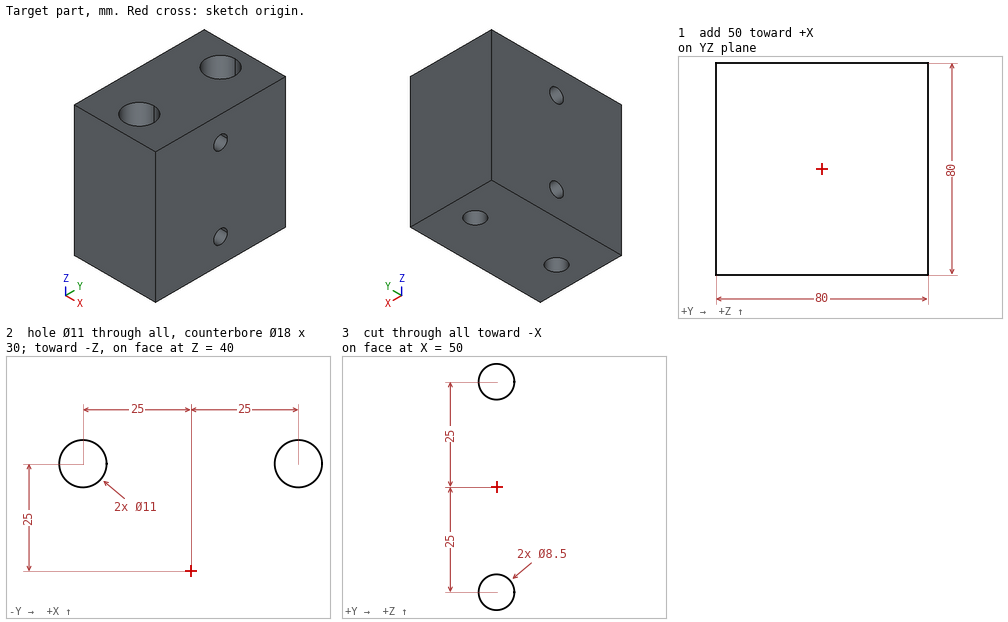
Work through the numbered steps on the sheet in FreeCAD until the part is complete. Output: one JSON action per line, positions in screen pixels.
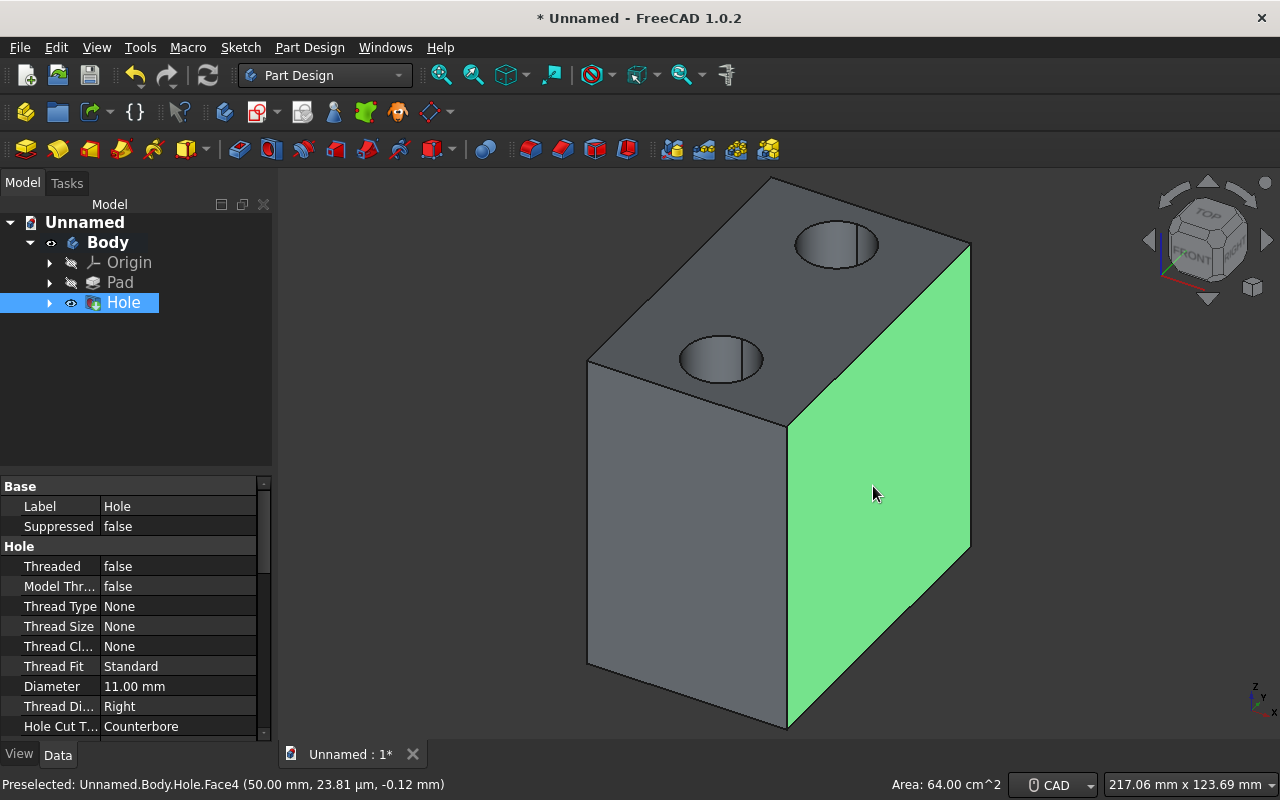
{"action": "left_click", "coordinate": [258, 112]}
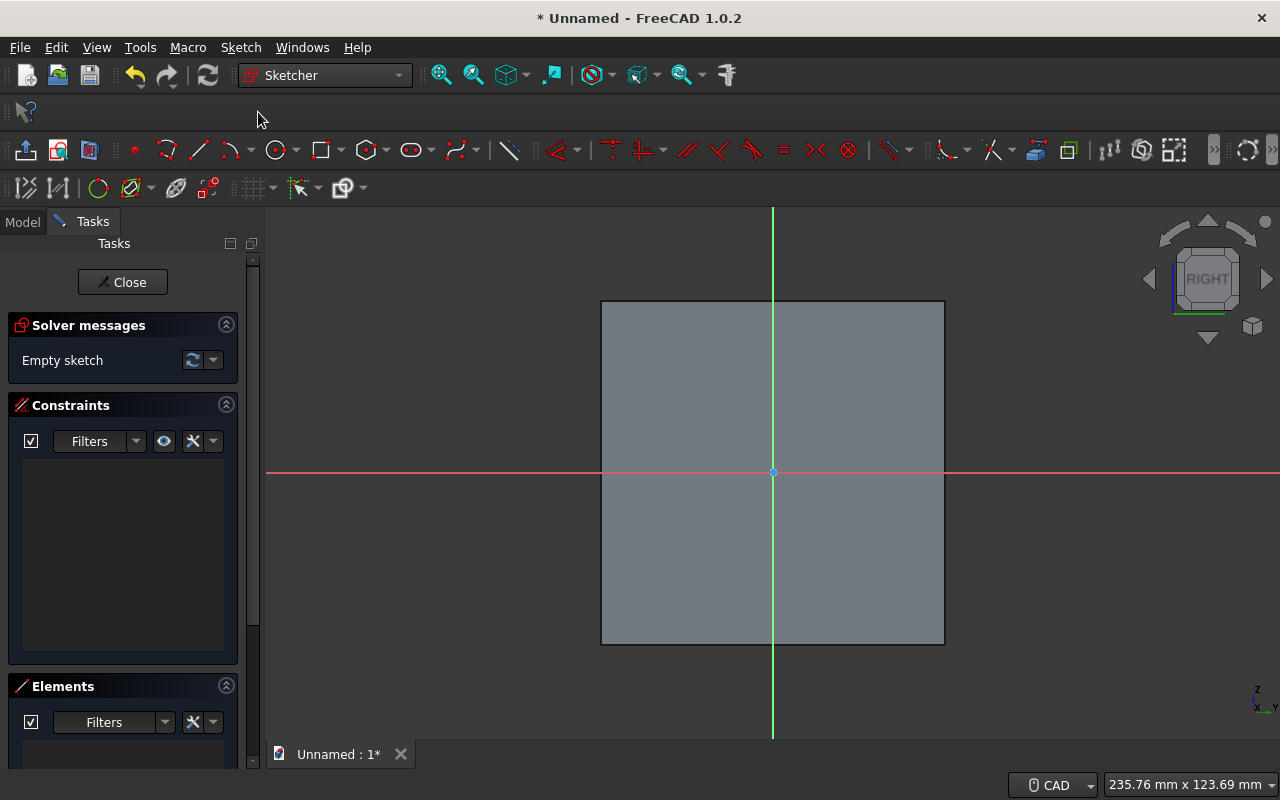
{"action": "left_click", "coordinate": [276, 150]}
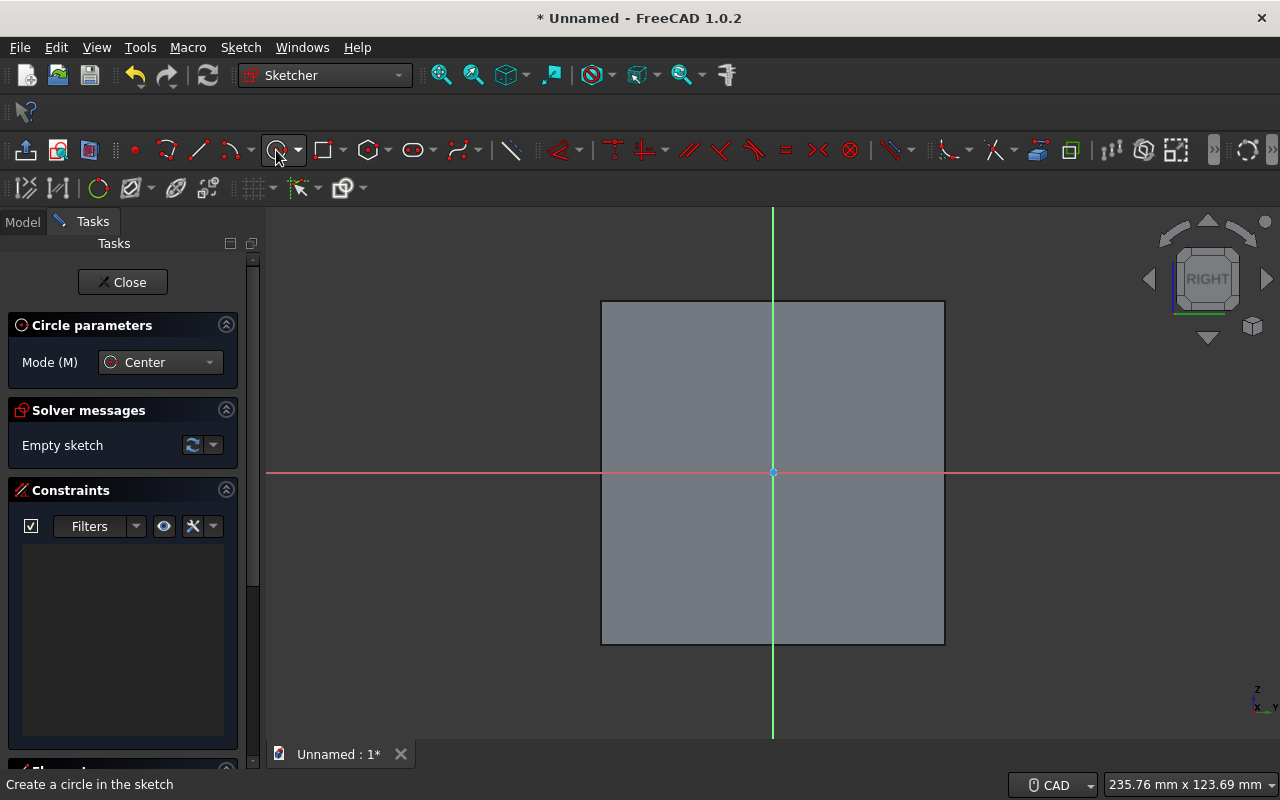
{"action": "scroll", "coordinate": [773, 581], "scroll_direction": "up", "scroll_amount": 2}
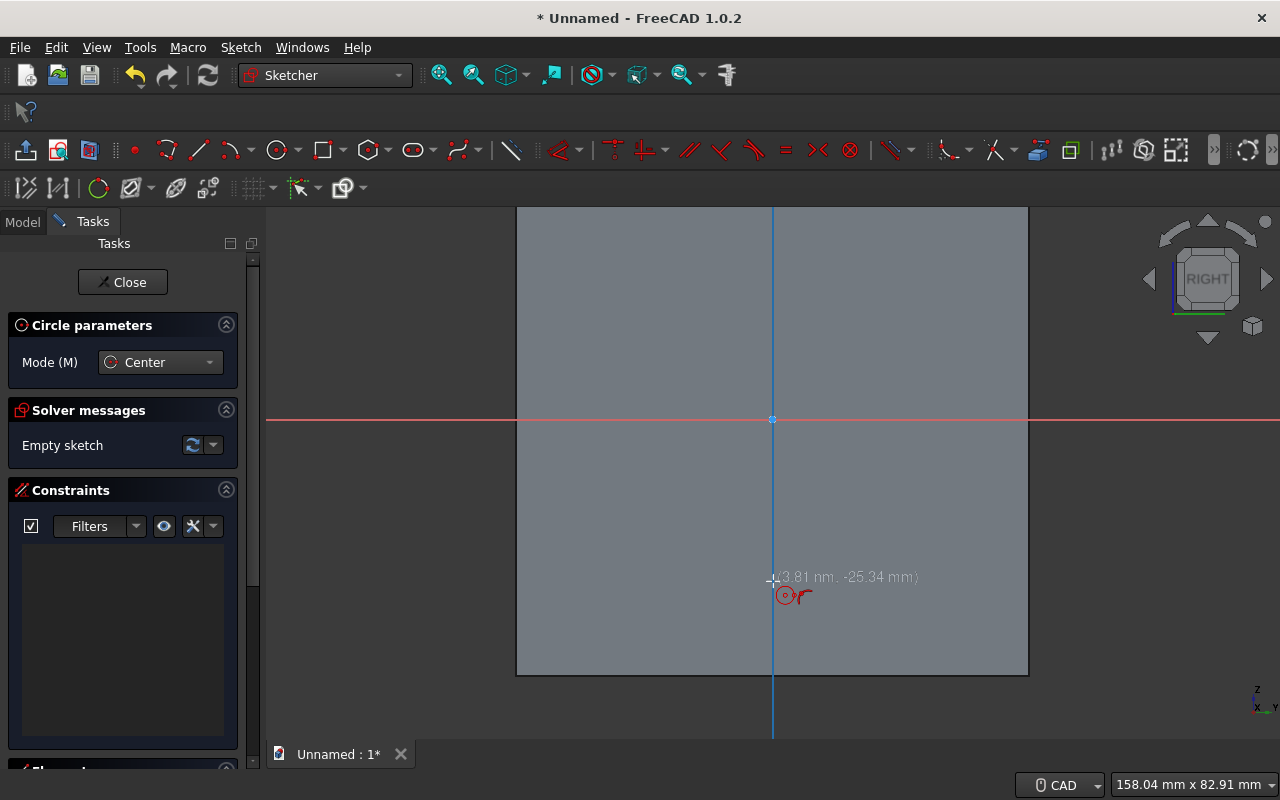
{"action": "left_click", "coordinate": [773, 580]}
{"action": "left_click", "coordinate": [792, 561]}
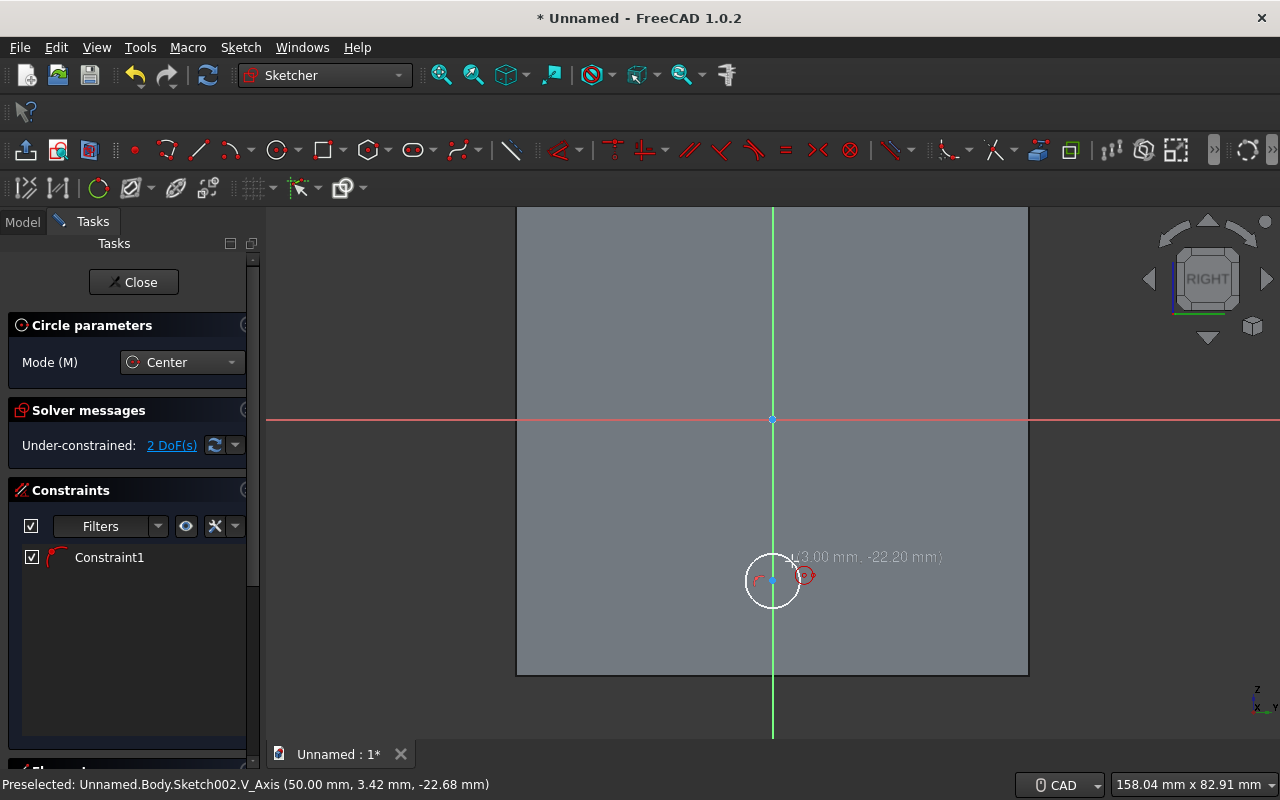
{"action": "left_click", "coordinate": [773, 259]}
{"action": "left_click", "coordinate": [792, 240]}
{"action": "key", "text": "Escape"}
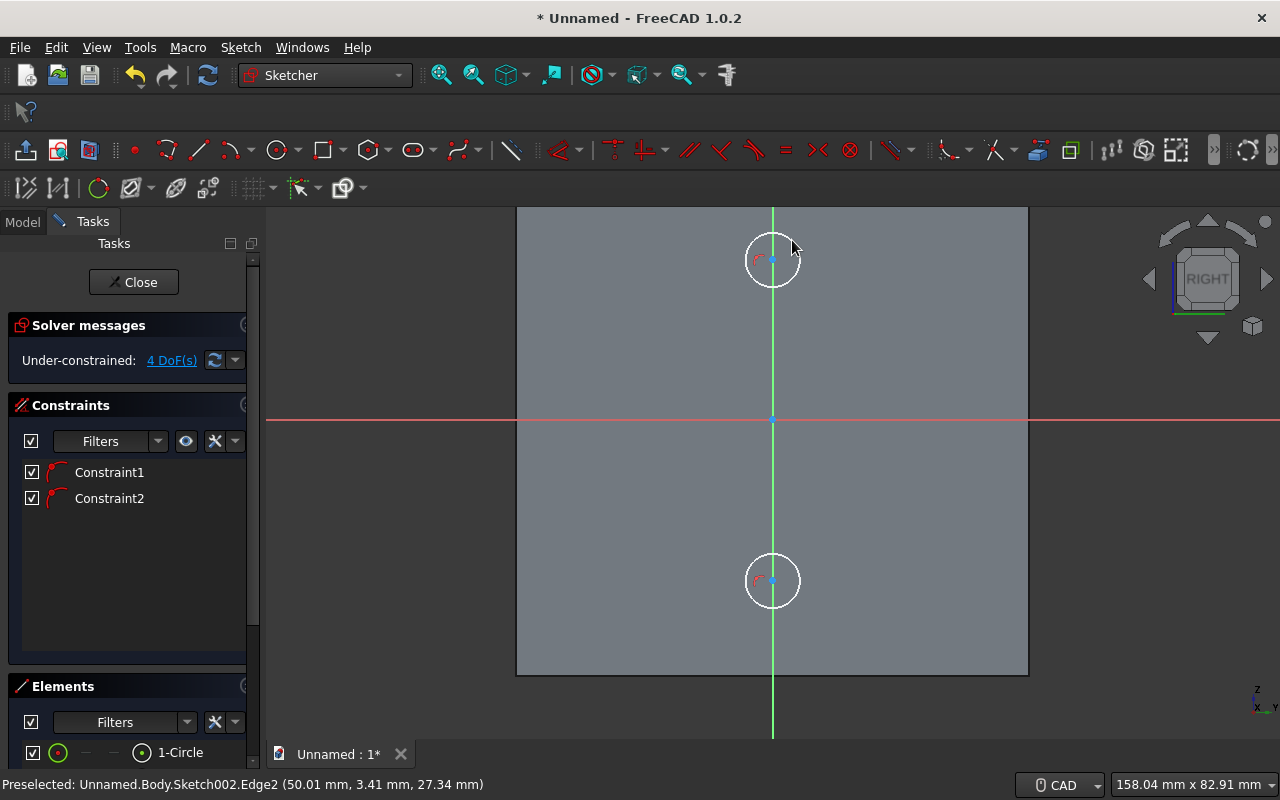
{"action": "left_click", "coordinate": [792, 562]}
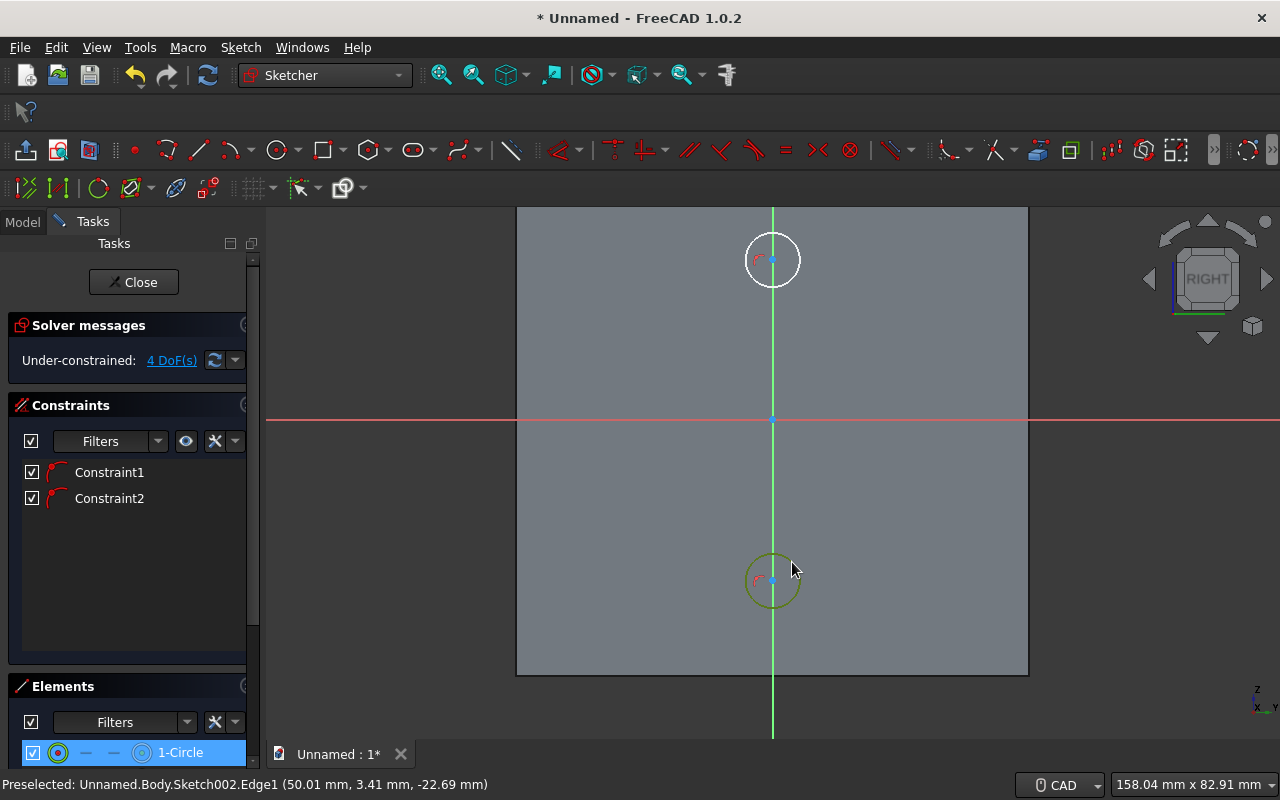
{"action": "left_click", "coordinate": [792, 241]}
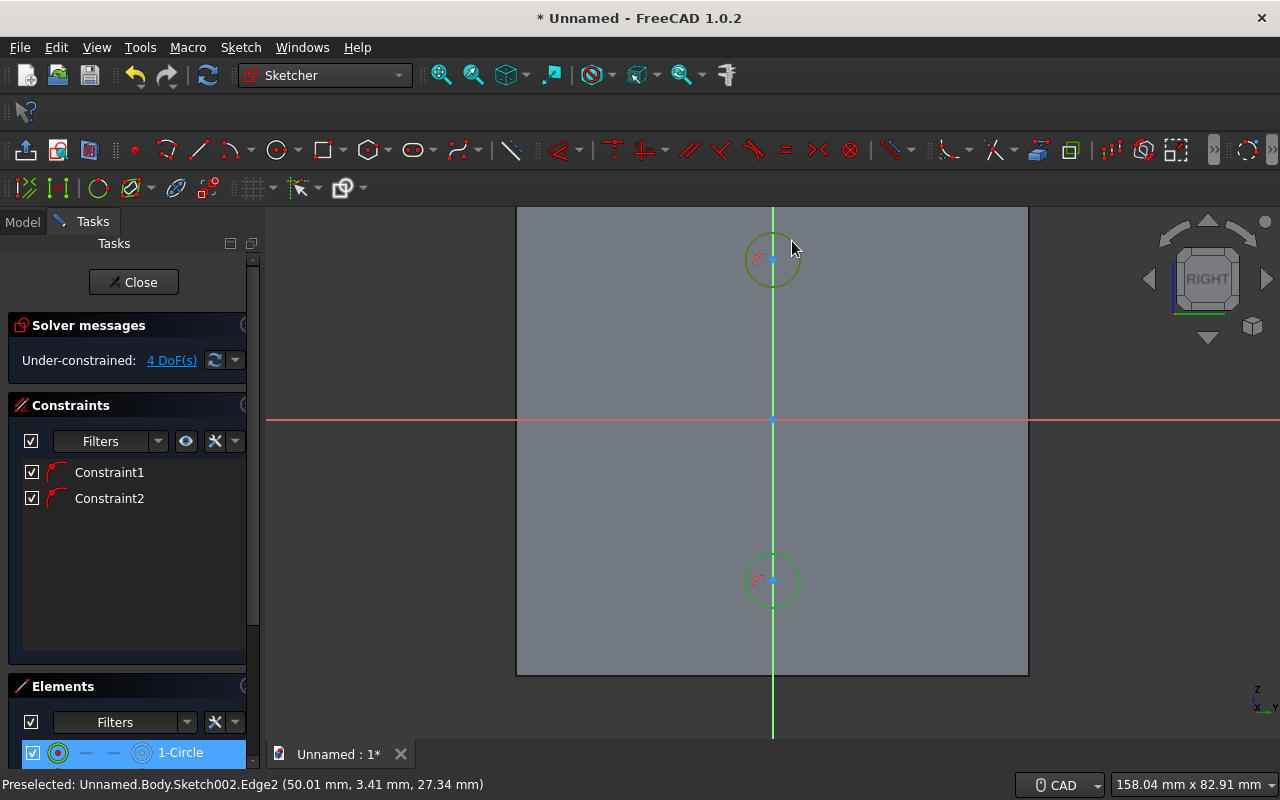
{"action": "left_click", "coordinate": [786, 150]}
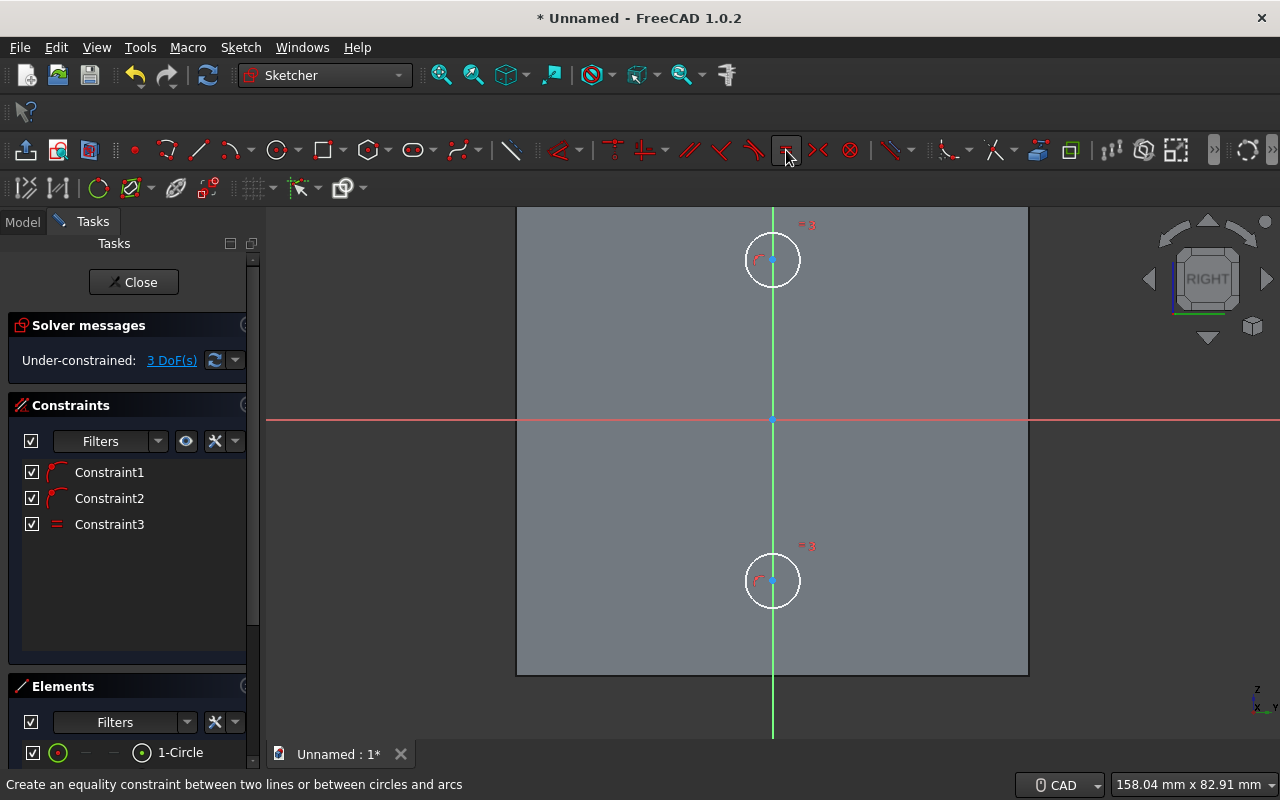
{"action": "left_click", "coordinate": [558, 150]}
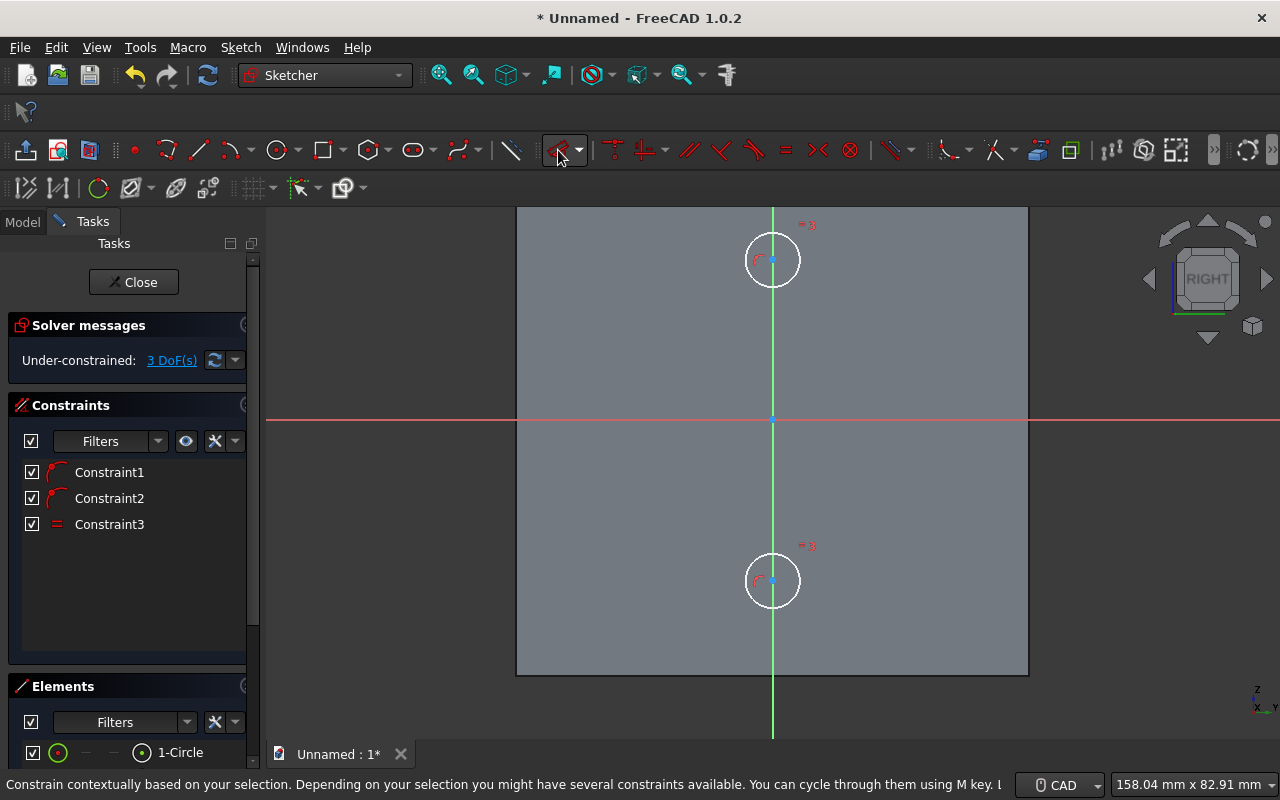
{"action": "left_click", "coordinate": [792, 562]}
{"action": "left_click", "coordinate": [815, 540]}